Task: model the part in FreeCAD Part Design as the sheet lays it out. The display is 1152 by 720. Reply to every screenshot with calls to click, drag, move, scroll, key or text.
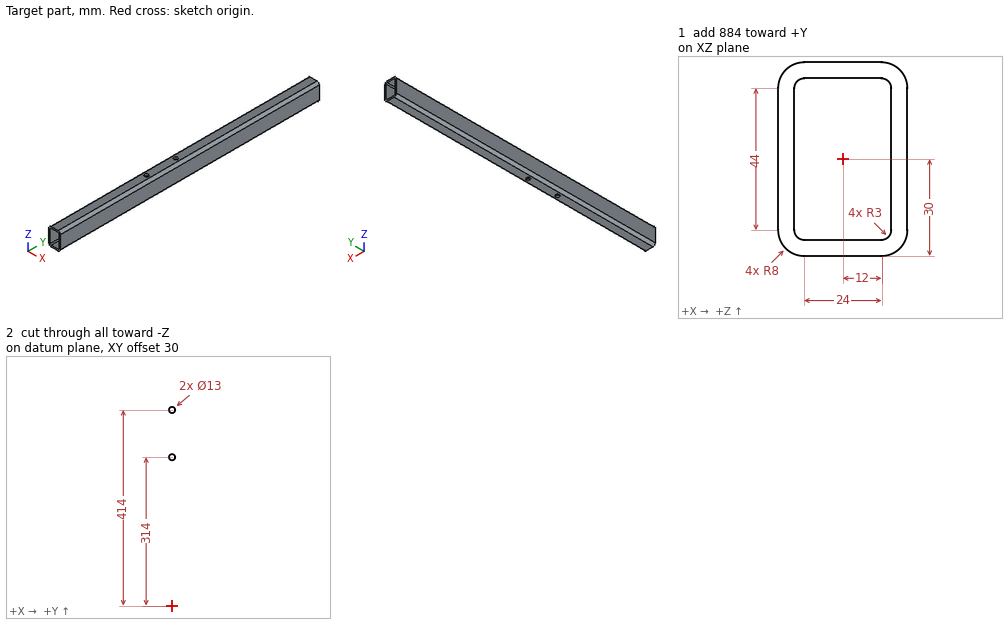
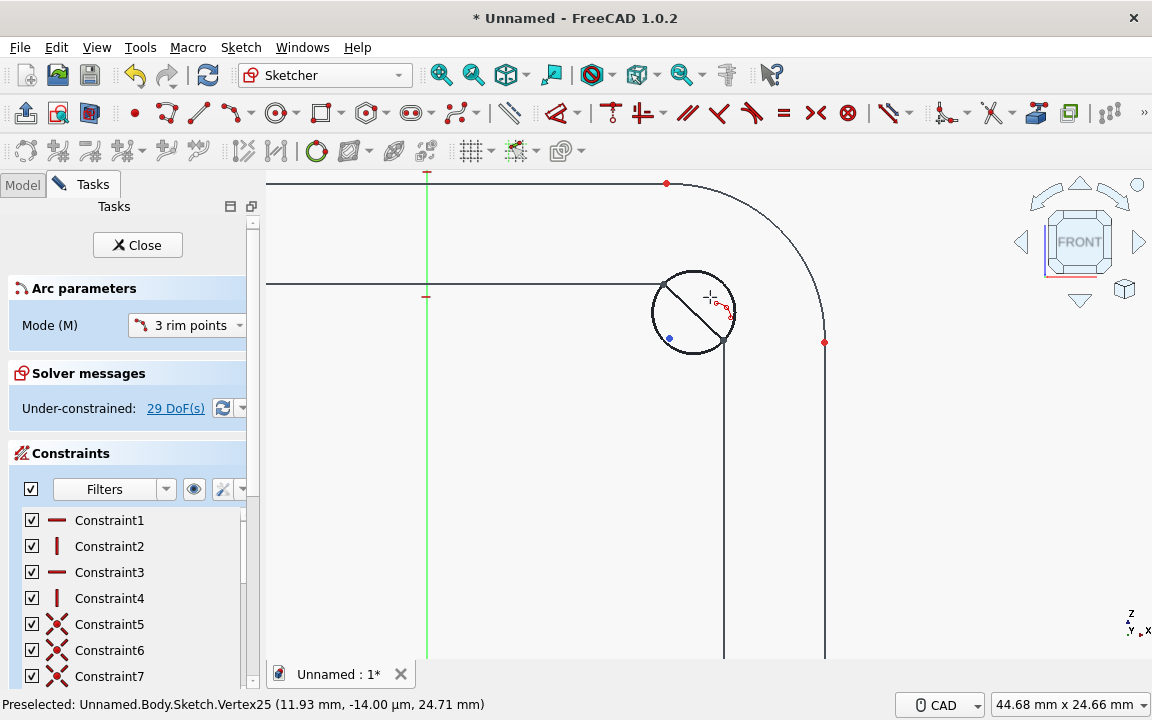
click(707, 296)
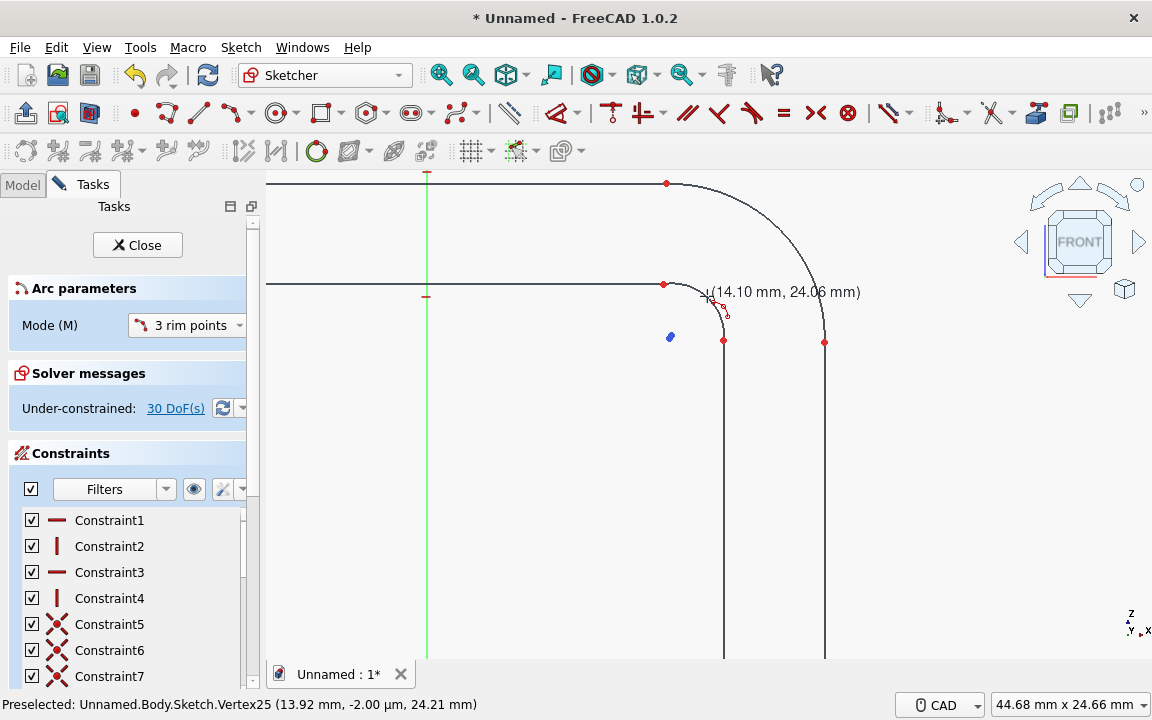
scroll(710, 297, down, 7)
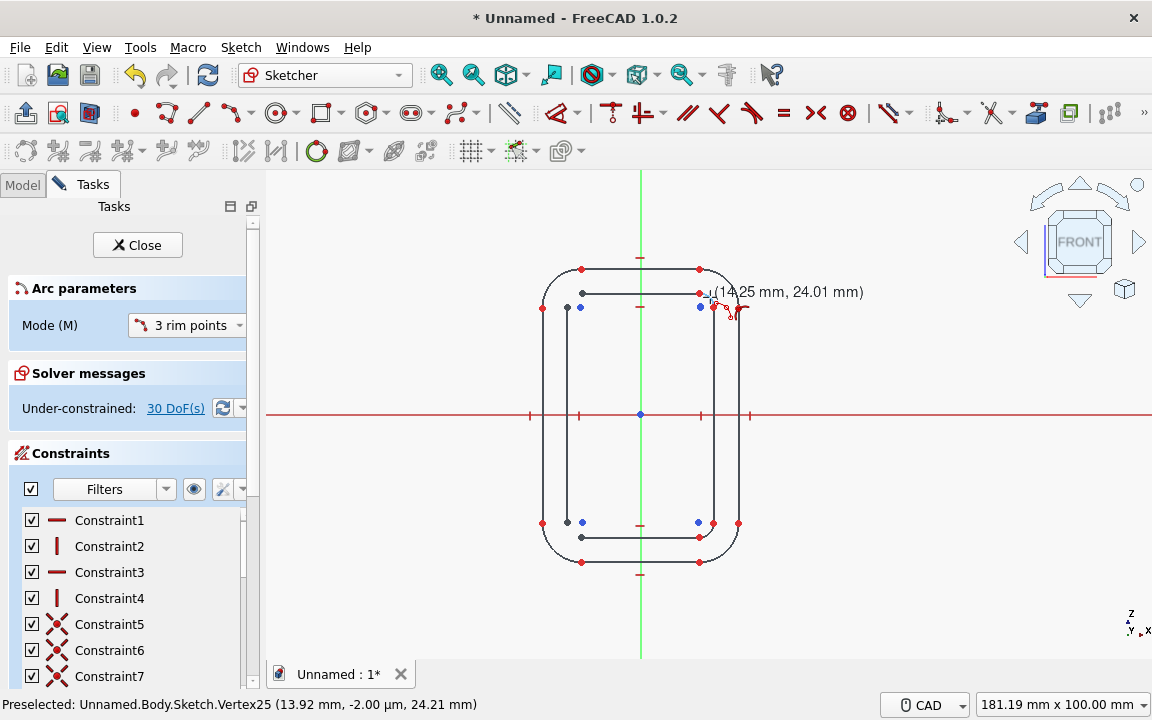
click(582, 294)
click(567, 308)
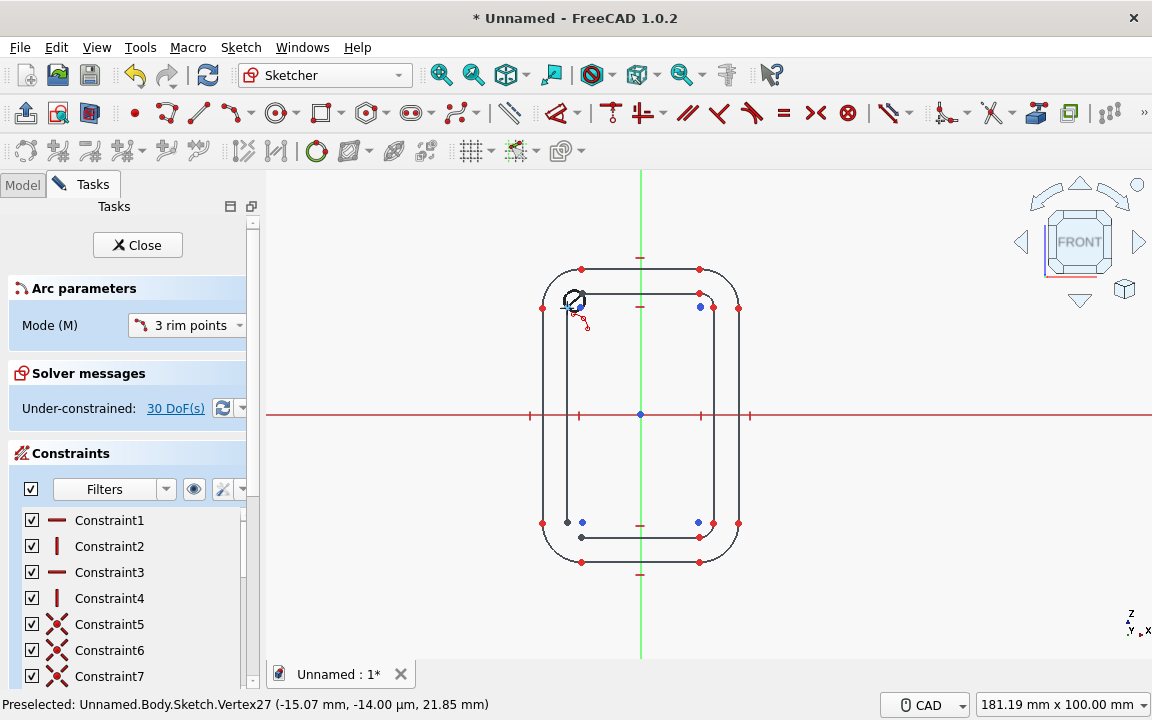
scroll(572, 297, up, 7)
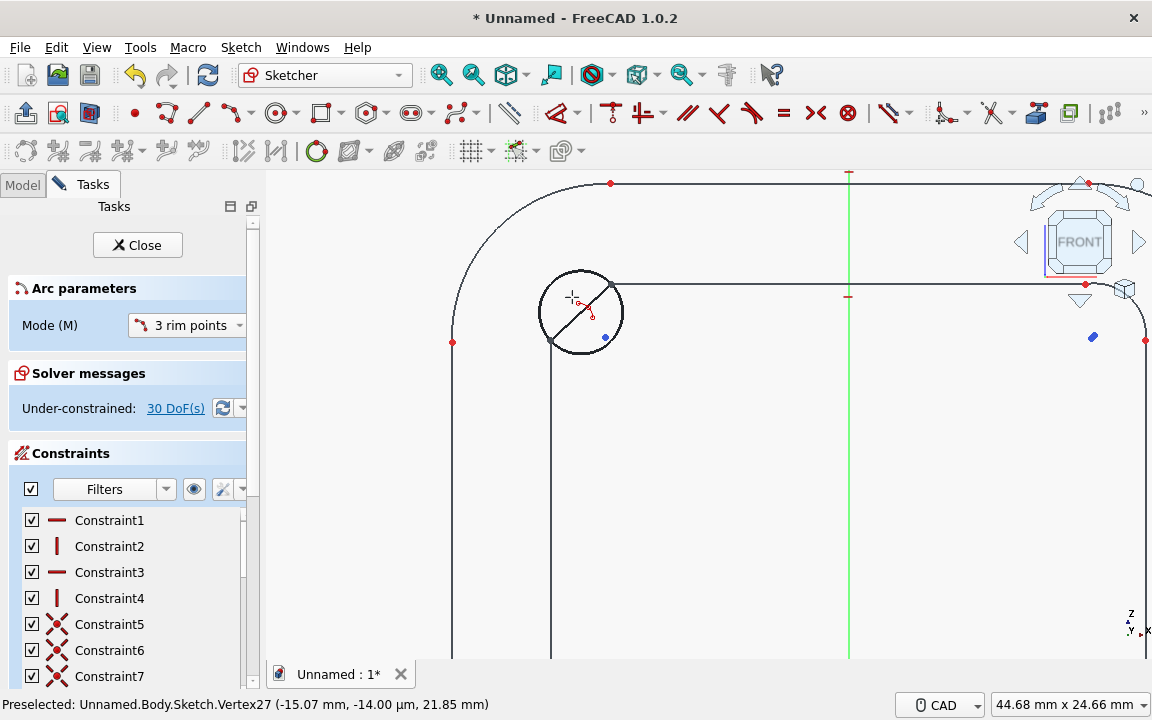
click(569, 296)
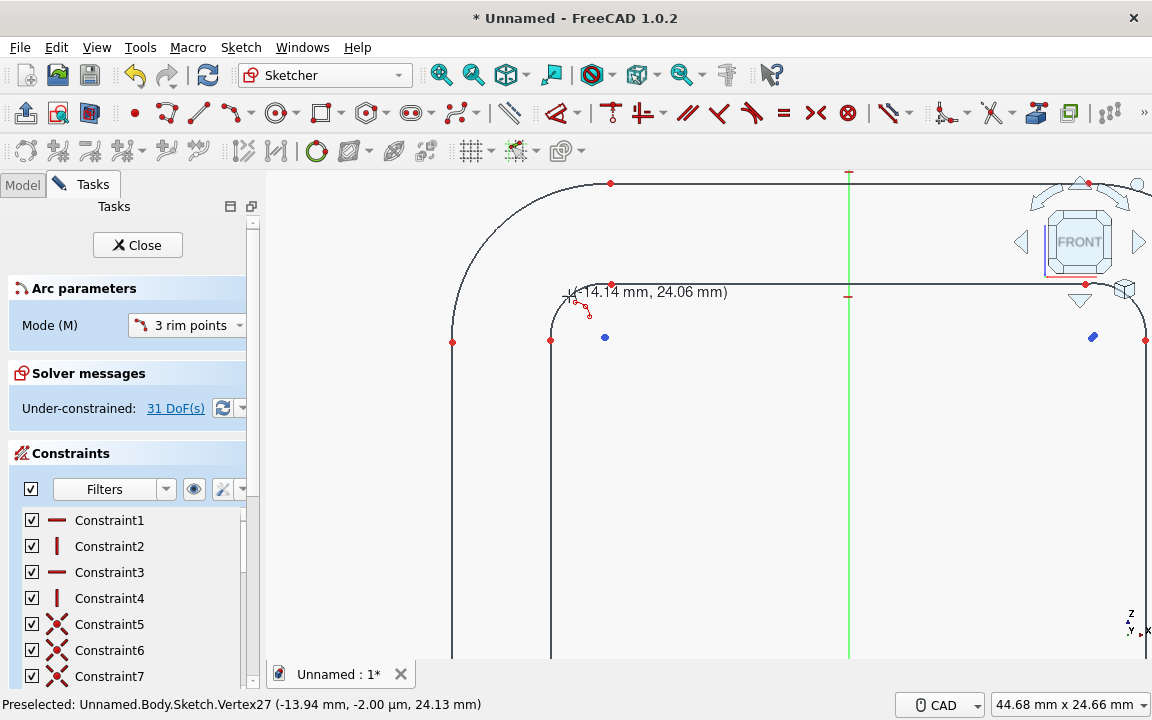
scroll(572, 297, down, 7)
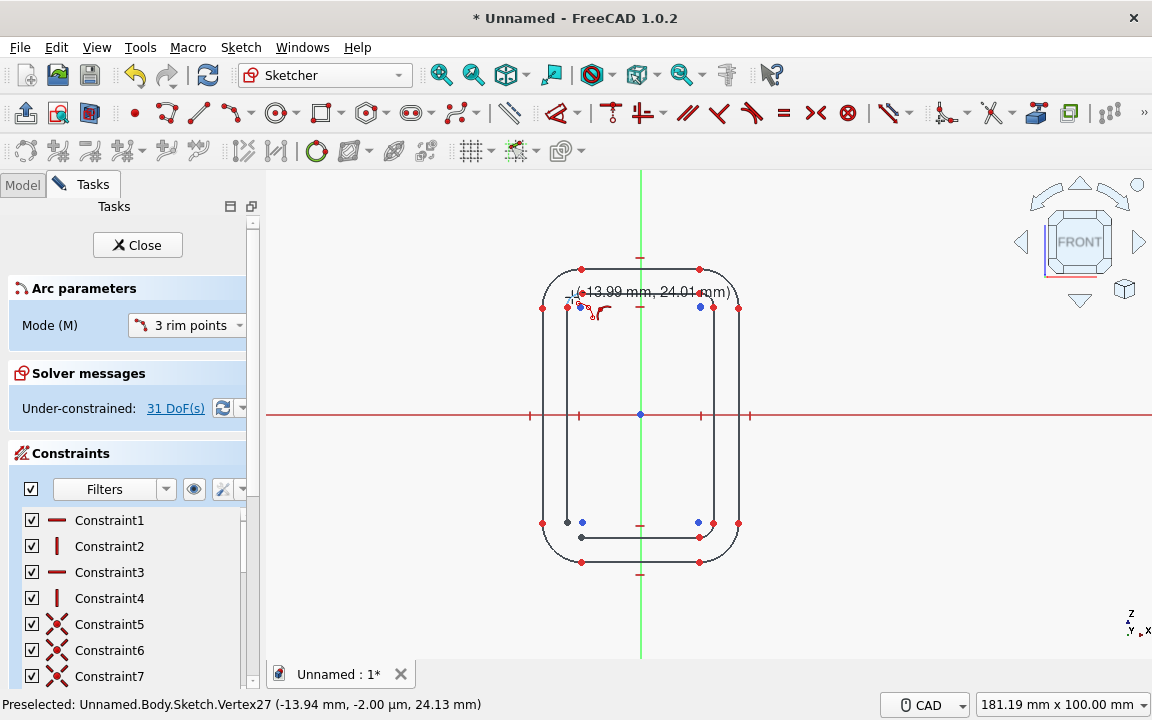
click(567, 523)
click(582, 538)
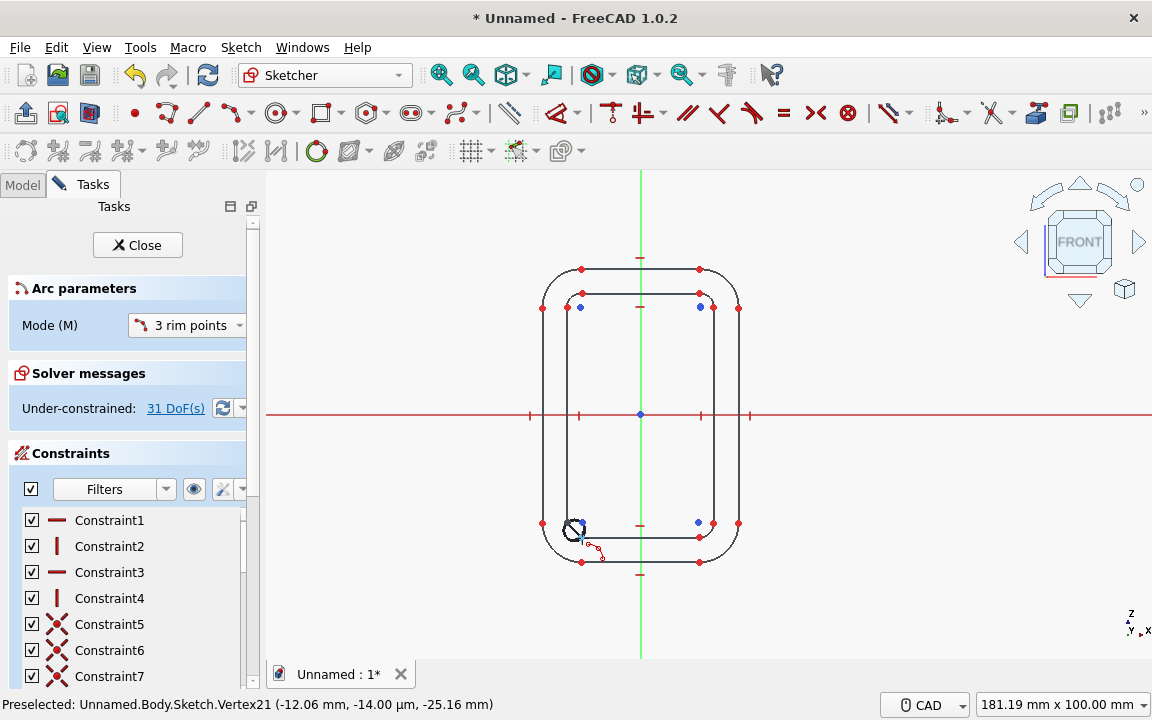
scroll(572, 533, up, 7)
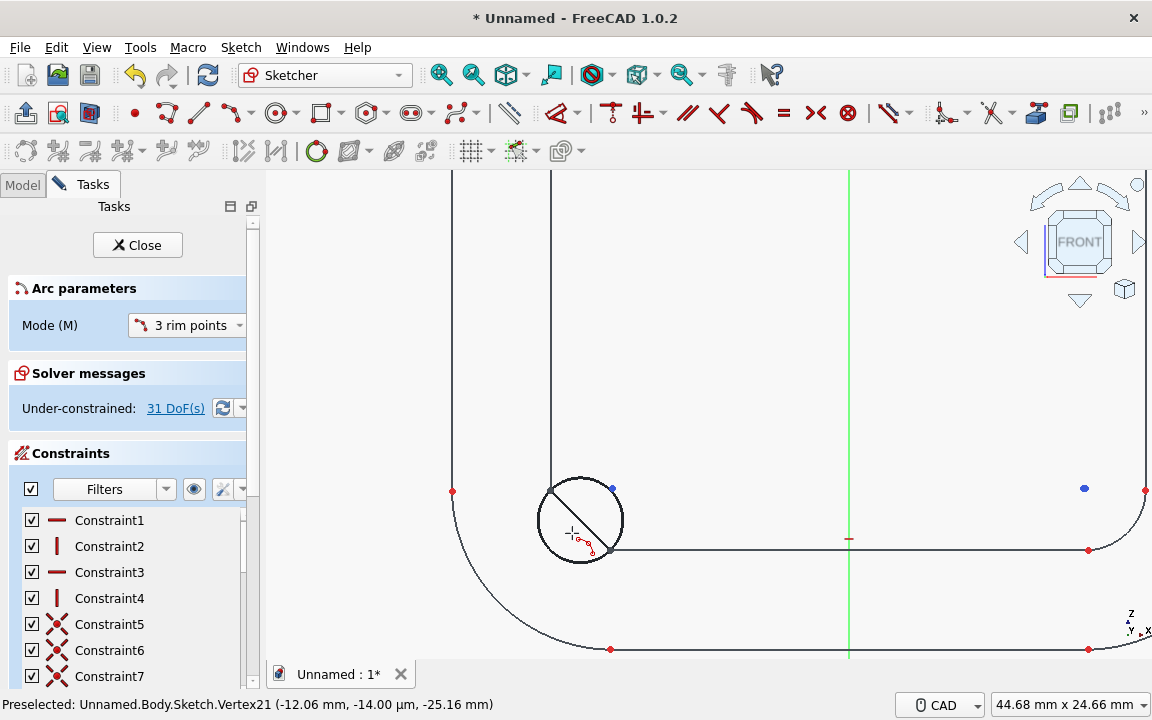
click(569, 530)
key(Escape)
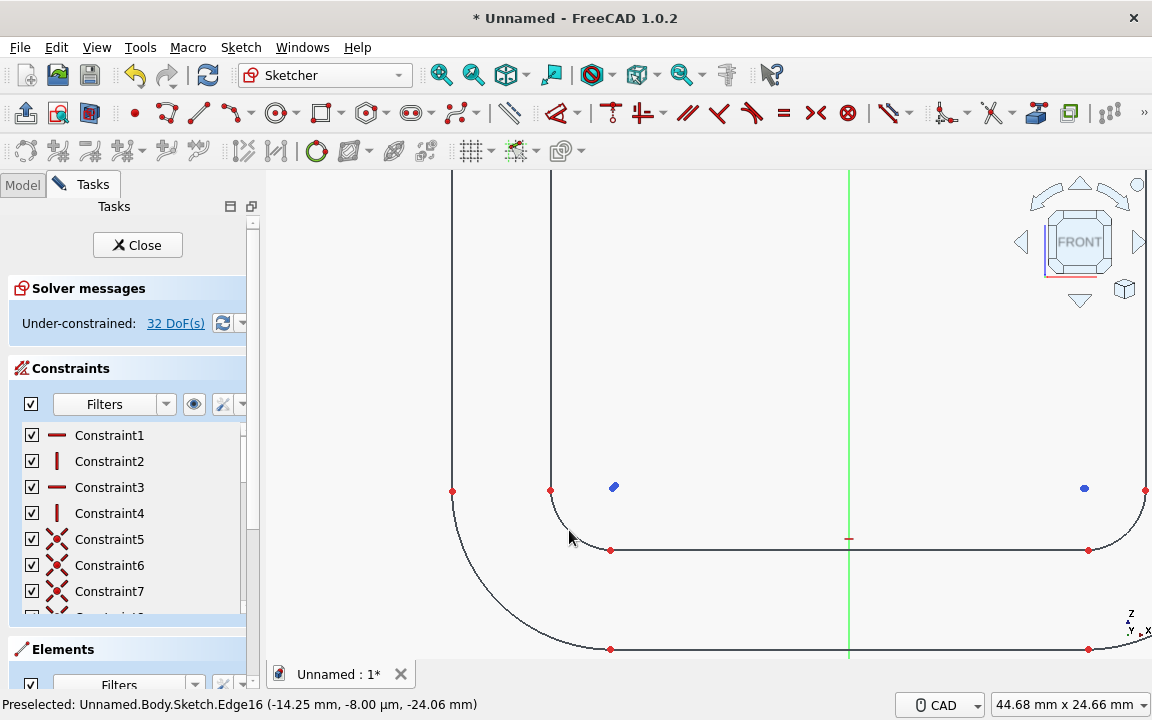
scroll(572, 533, down, 7)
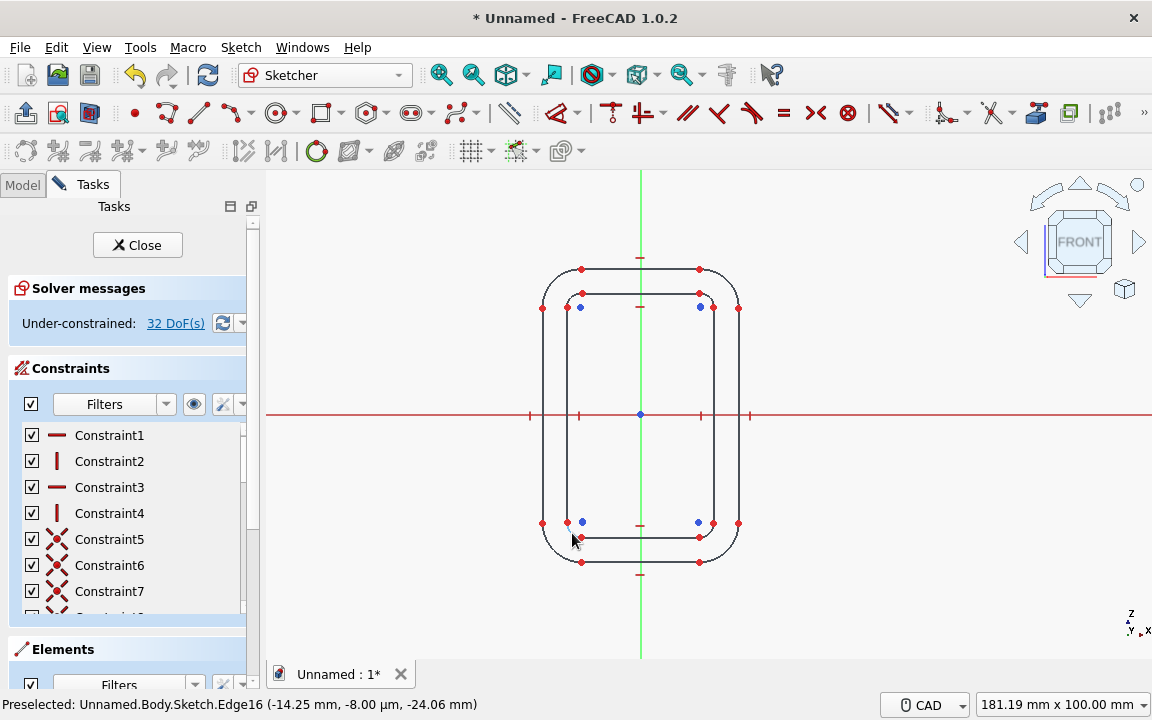
click(664, 562)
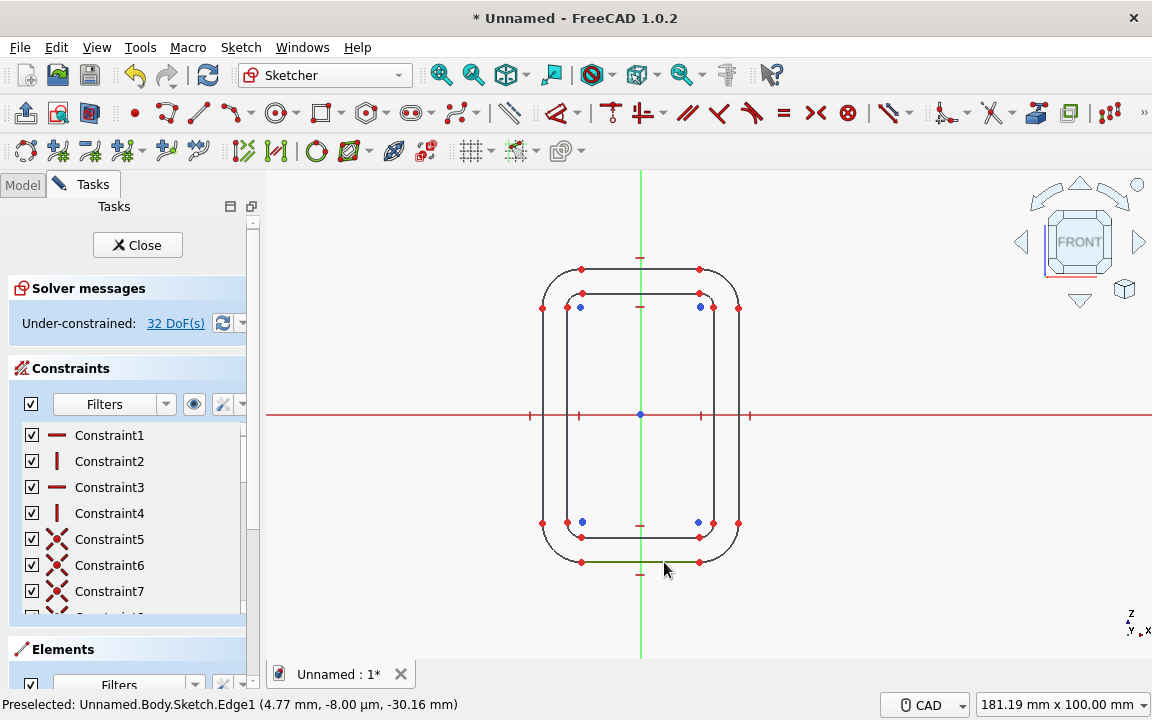
click(547, 541)